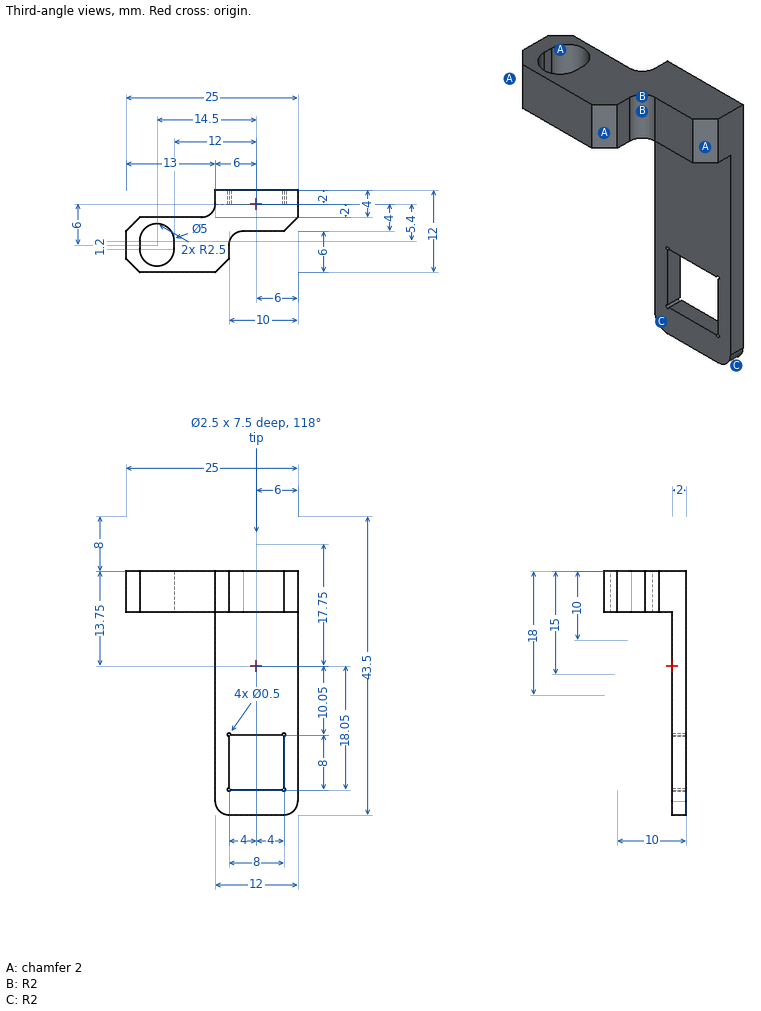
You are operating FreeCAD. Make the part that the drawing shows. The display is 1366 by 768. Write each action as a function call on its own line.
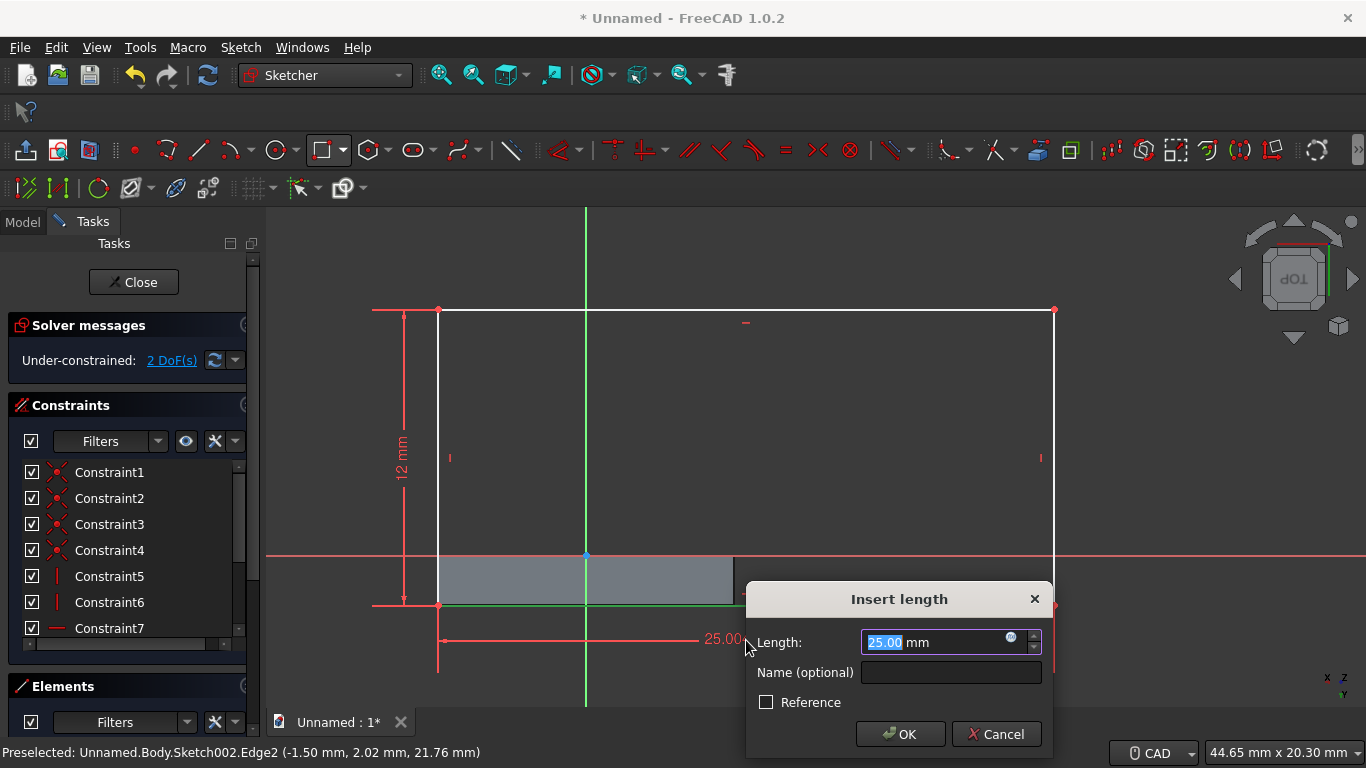
text(25)
key(Return)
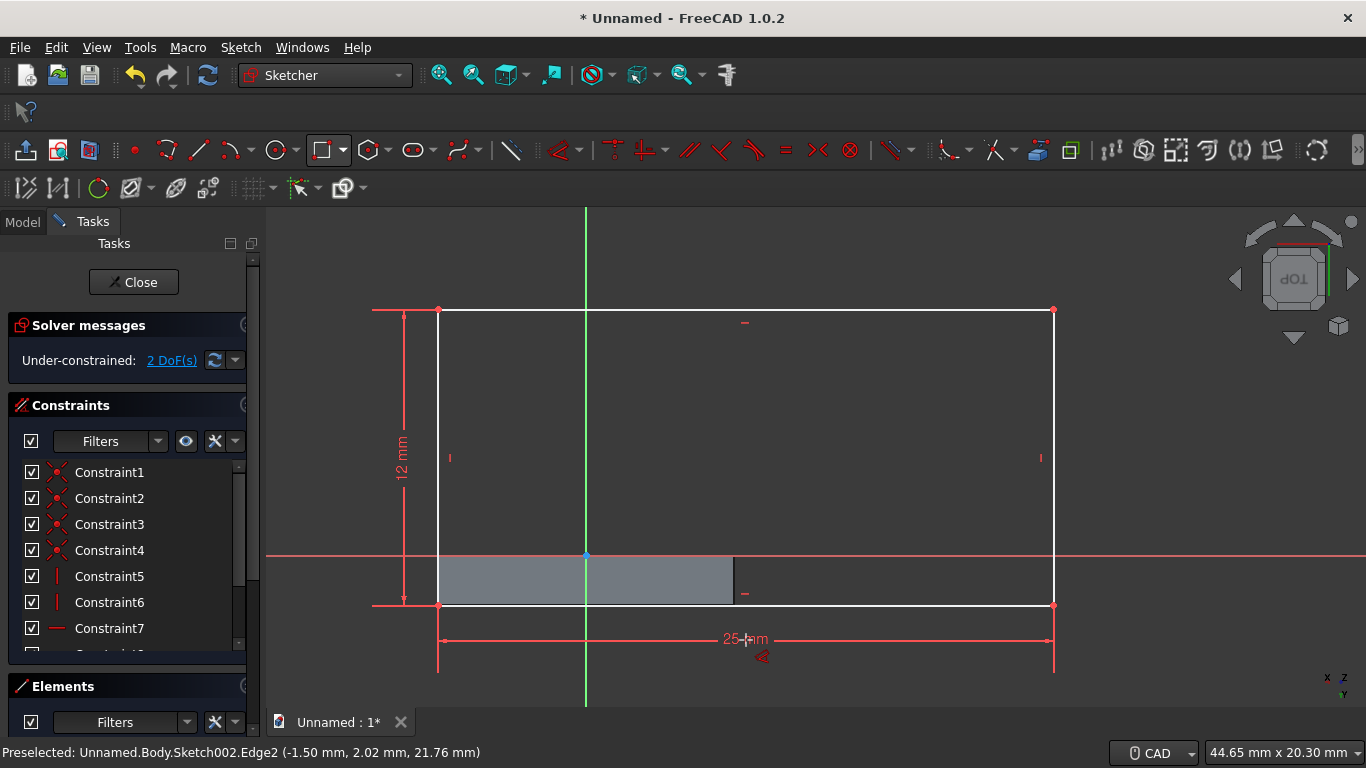
click(438, 310)
click(512, 276)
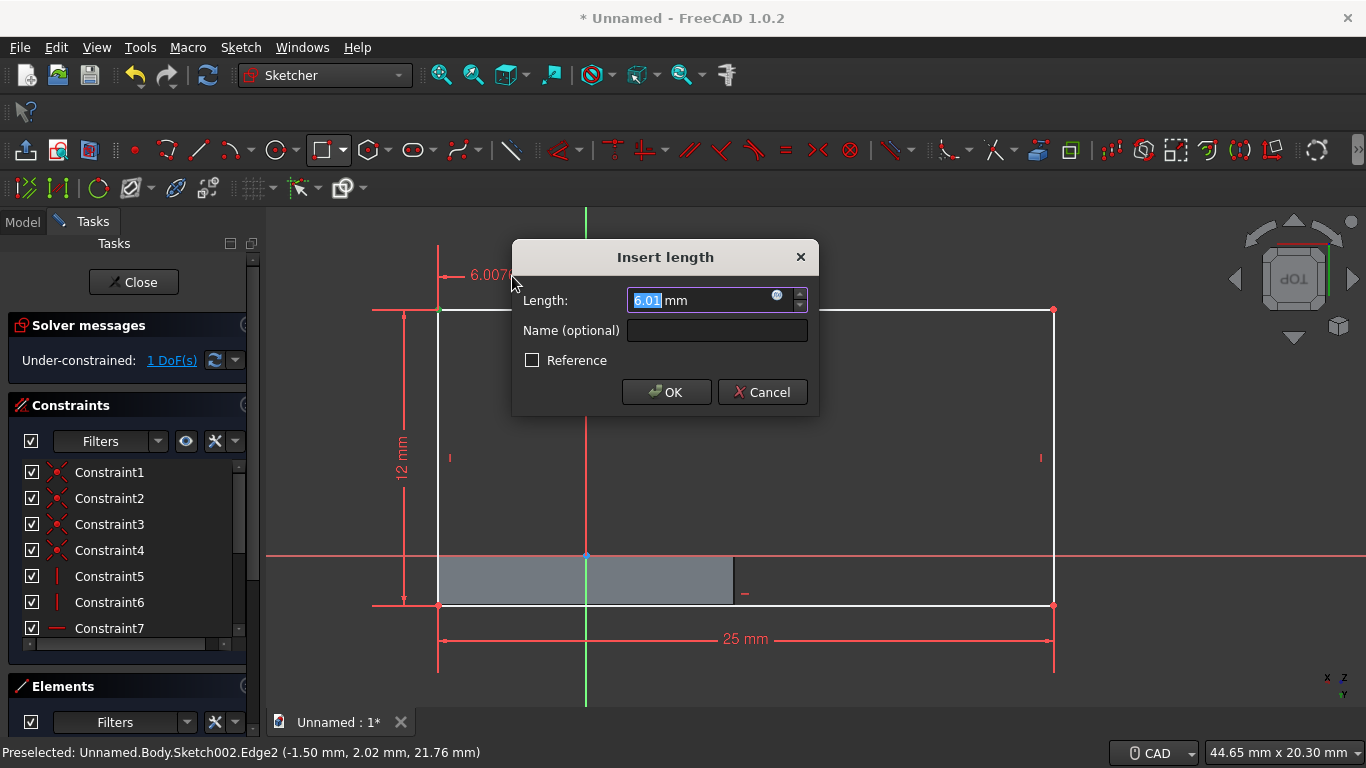
text(6)
key(Return)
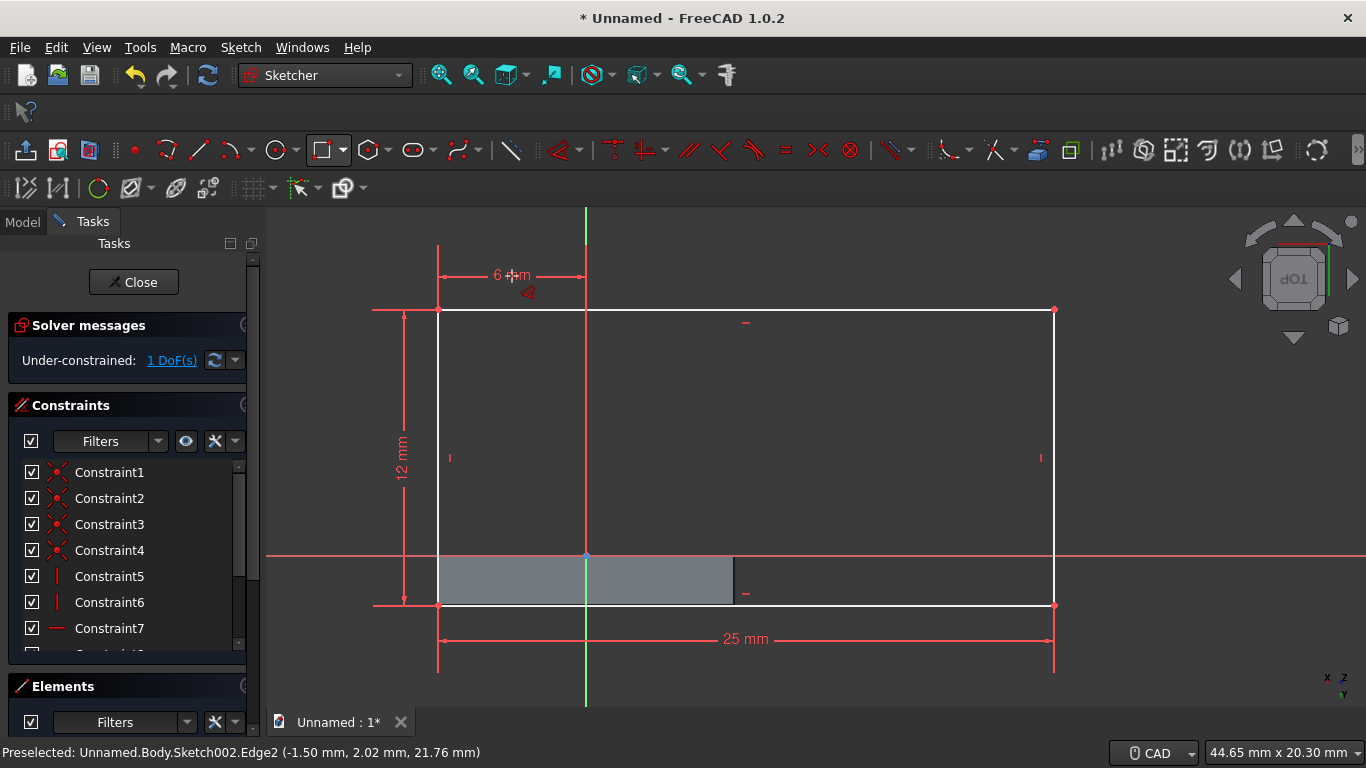
click(438, 606)
click(404, 581)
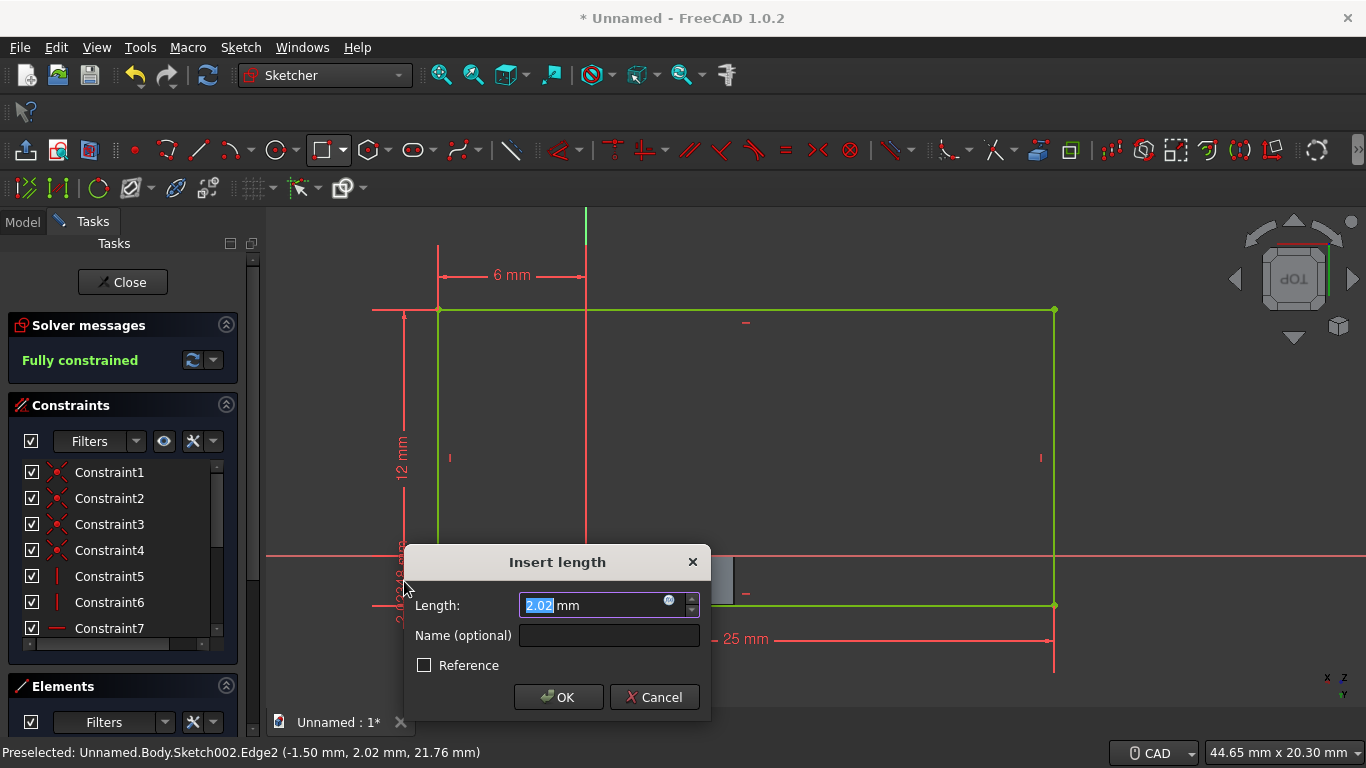
text(2)
key(Return)
key(Escape)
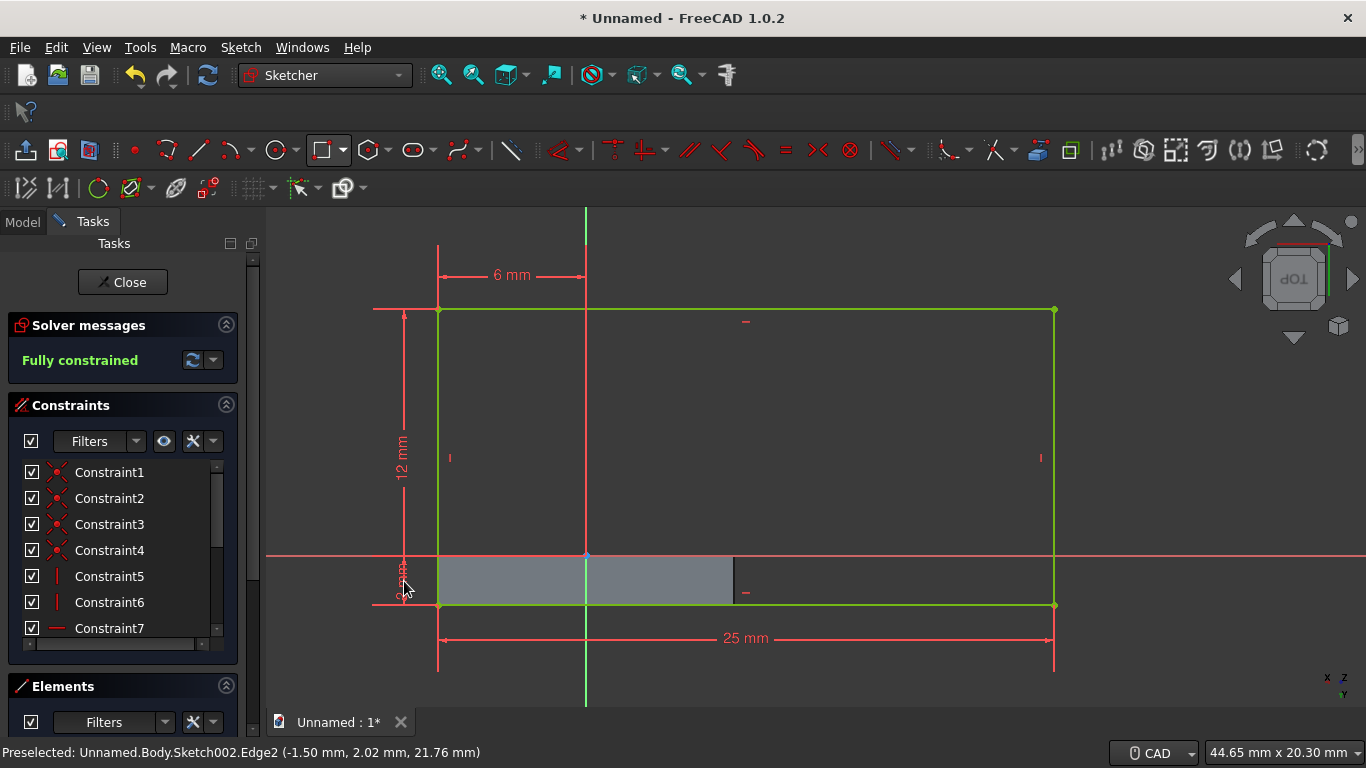
click(123, 282)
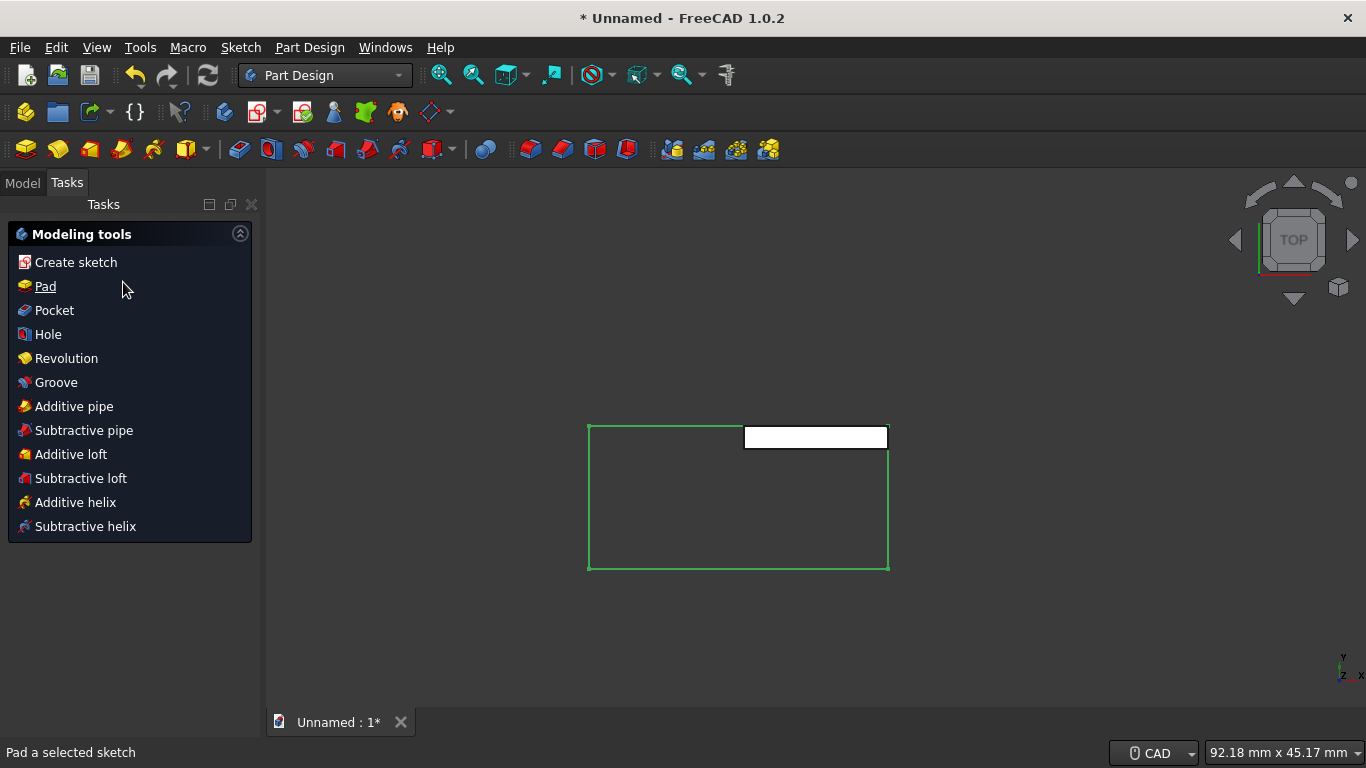
click(26, 150)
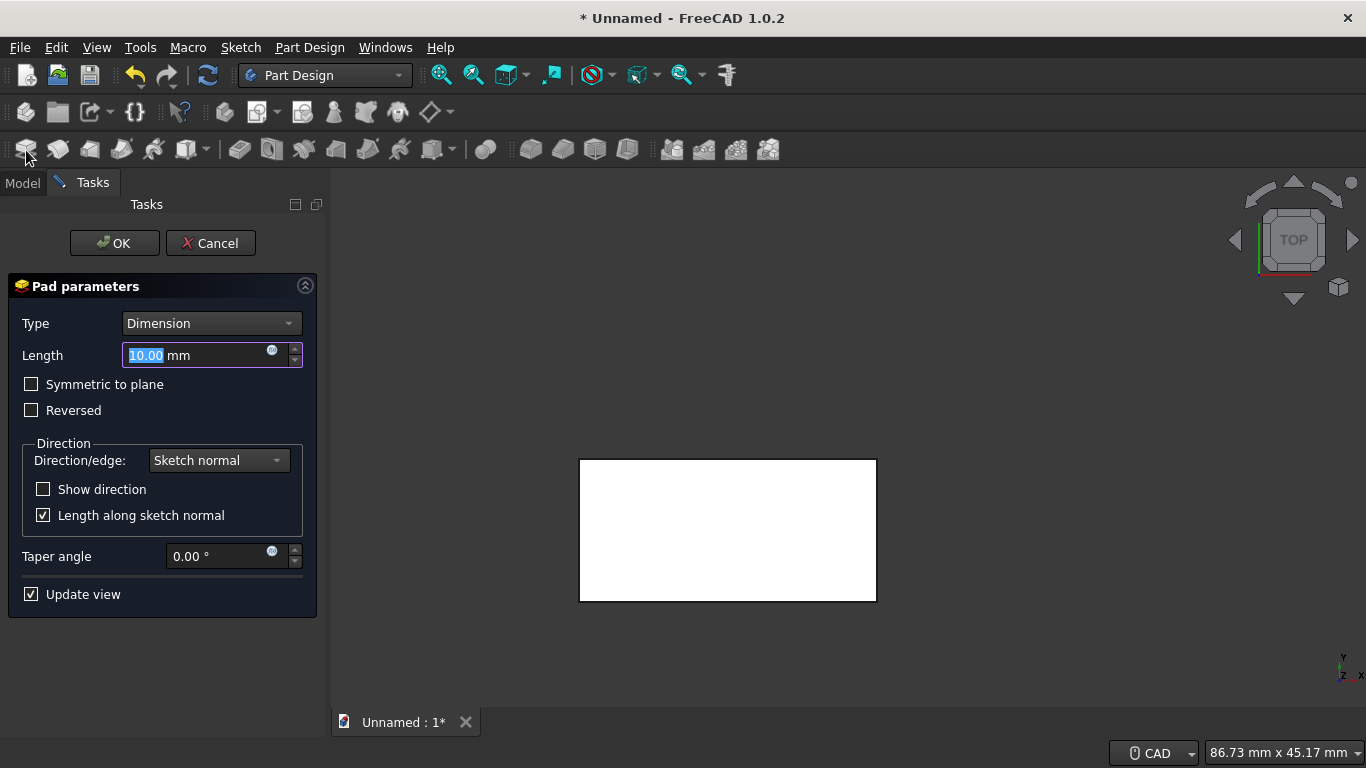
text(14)
key(Tab)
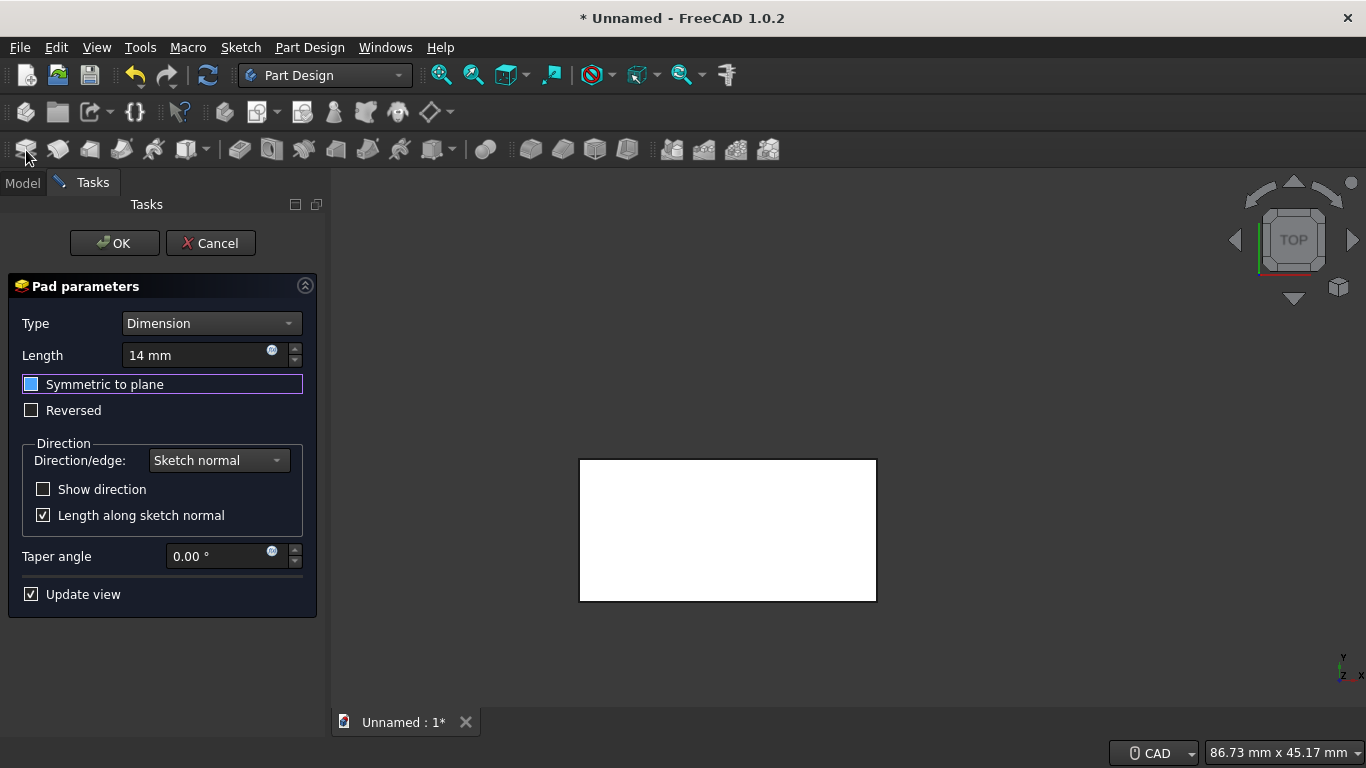
click(30, 410)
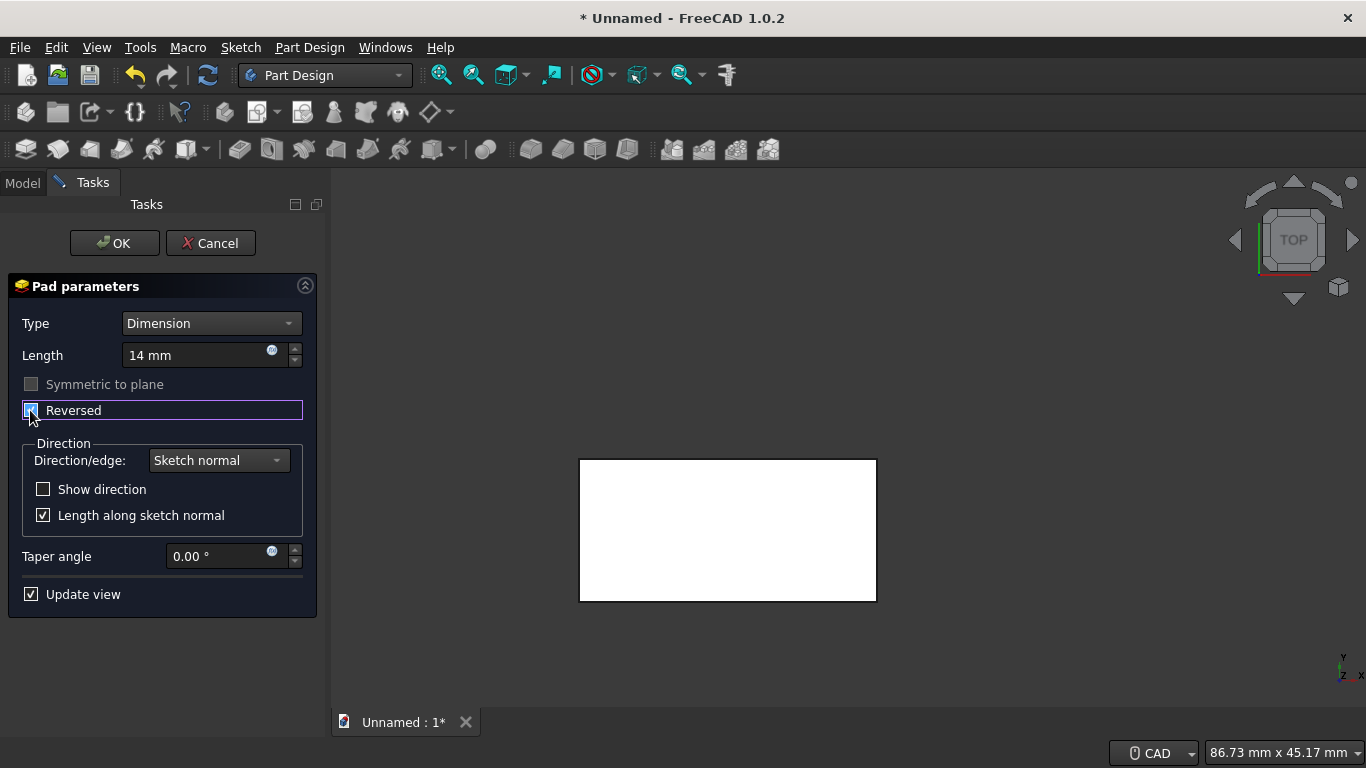
click(115, 243)